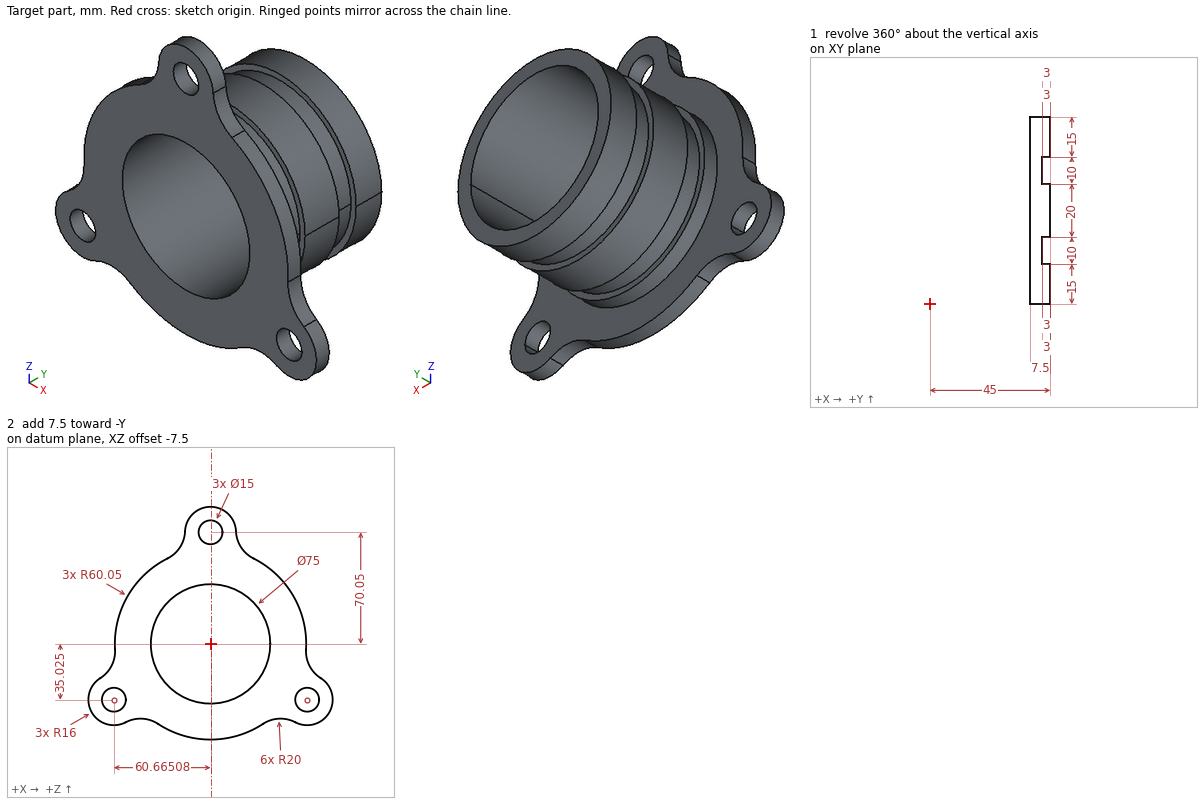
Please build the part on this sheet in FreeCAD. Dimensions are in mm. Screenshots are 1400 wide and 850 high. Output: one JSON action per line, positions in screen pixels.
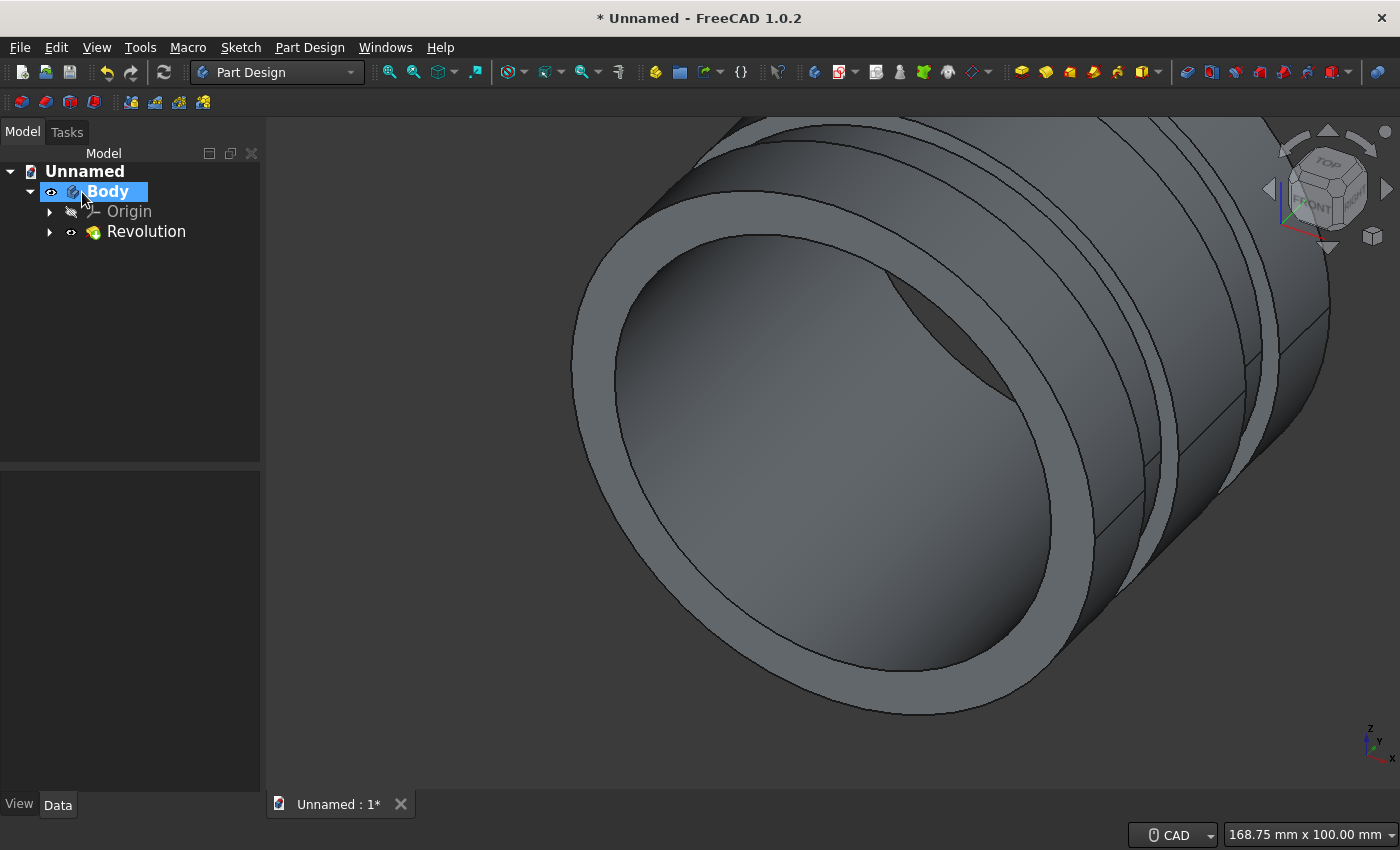
{"action": "left_click", "coordinate": [390, 72]}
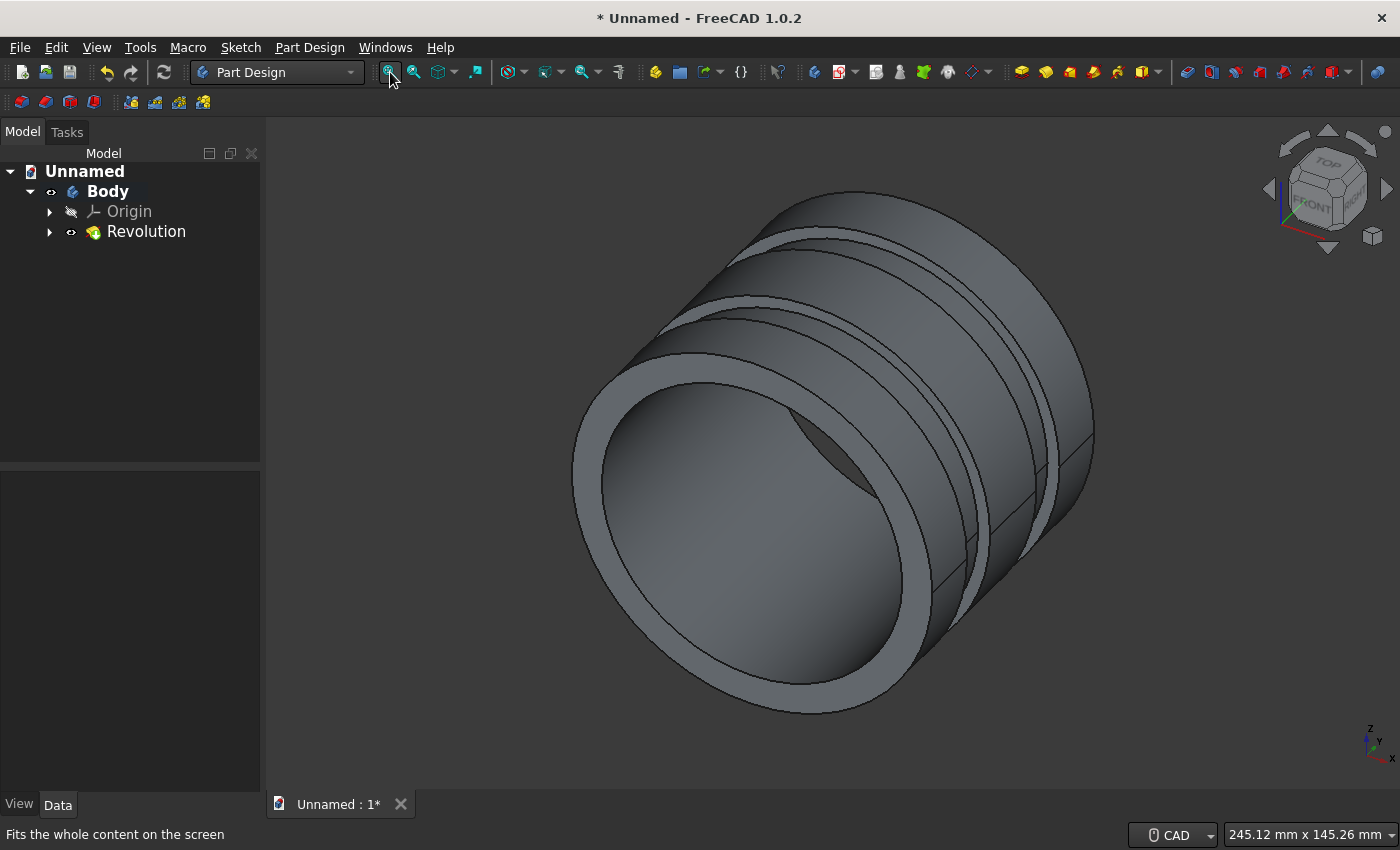
{"action": "left_click", "coordinate": [50, 212]}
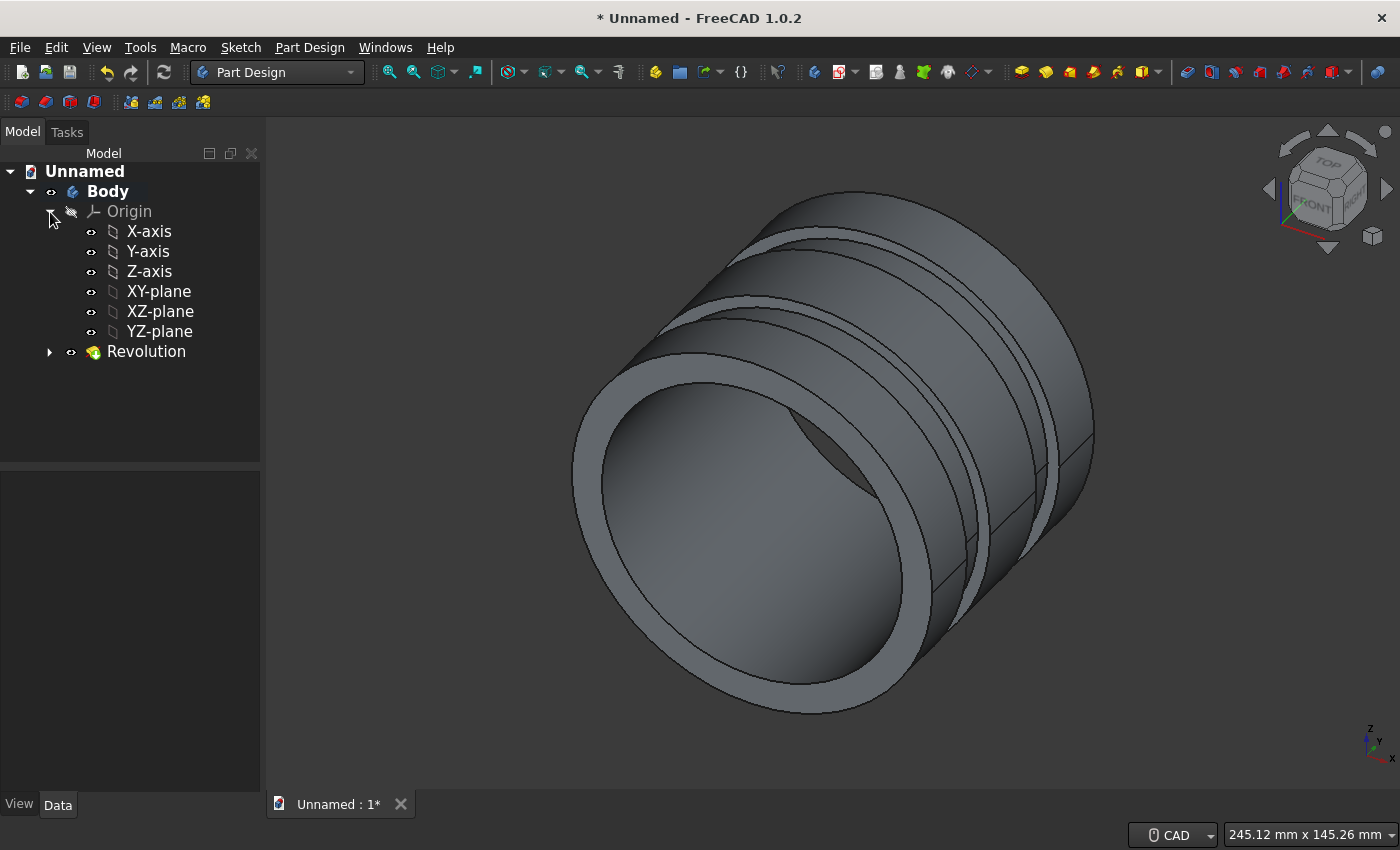
{"action": "left_click", "coordinate": [136, 312]}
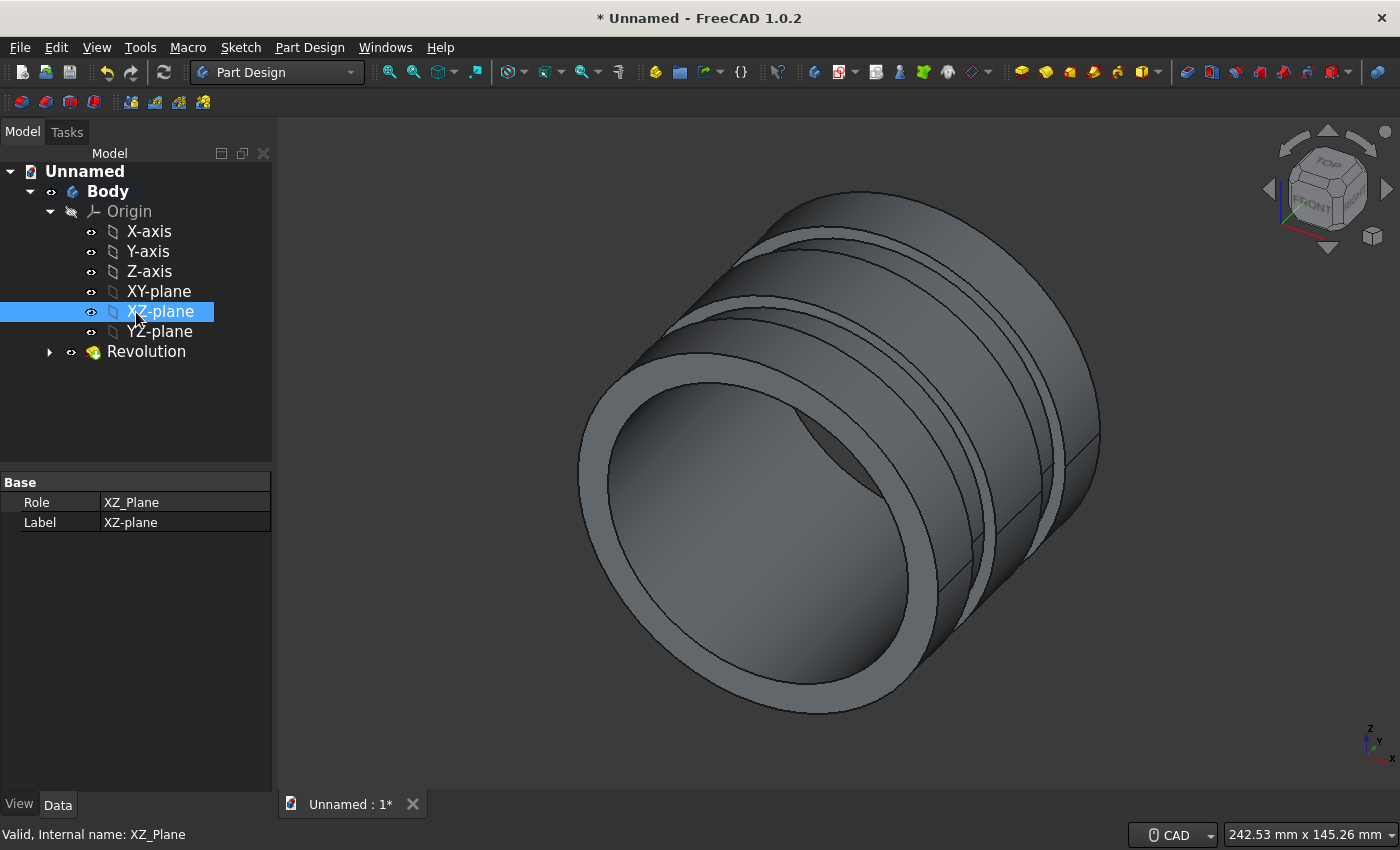
{"action": "left_click", "coordinate": [972, 72]}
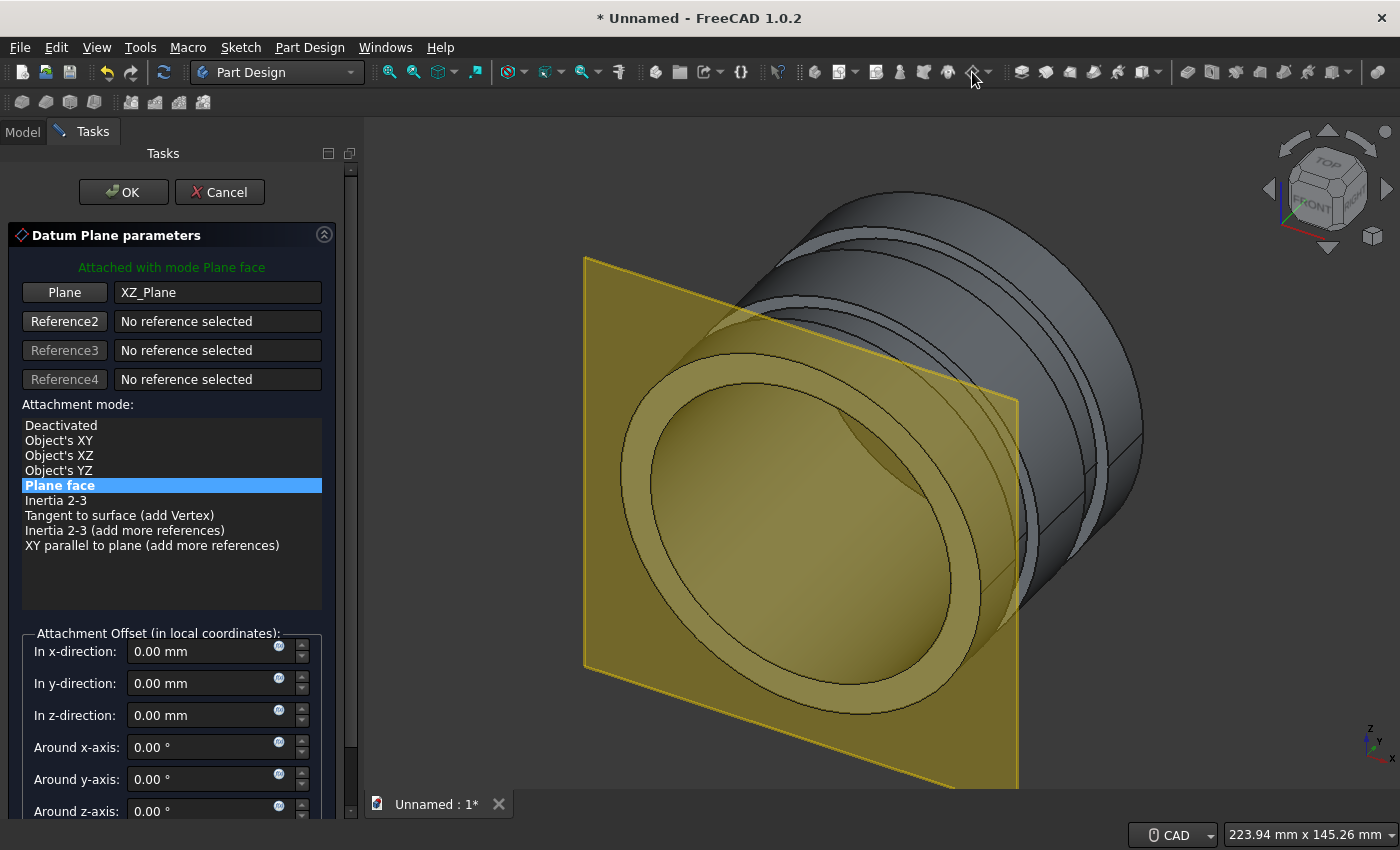
{"action": "triple_click", "coordinate": [210, 715]}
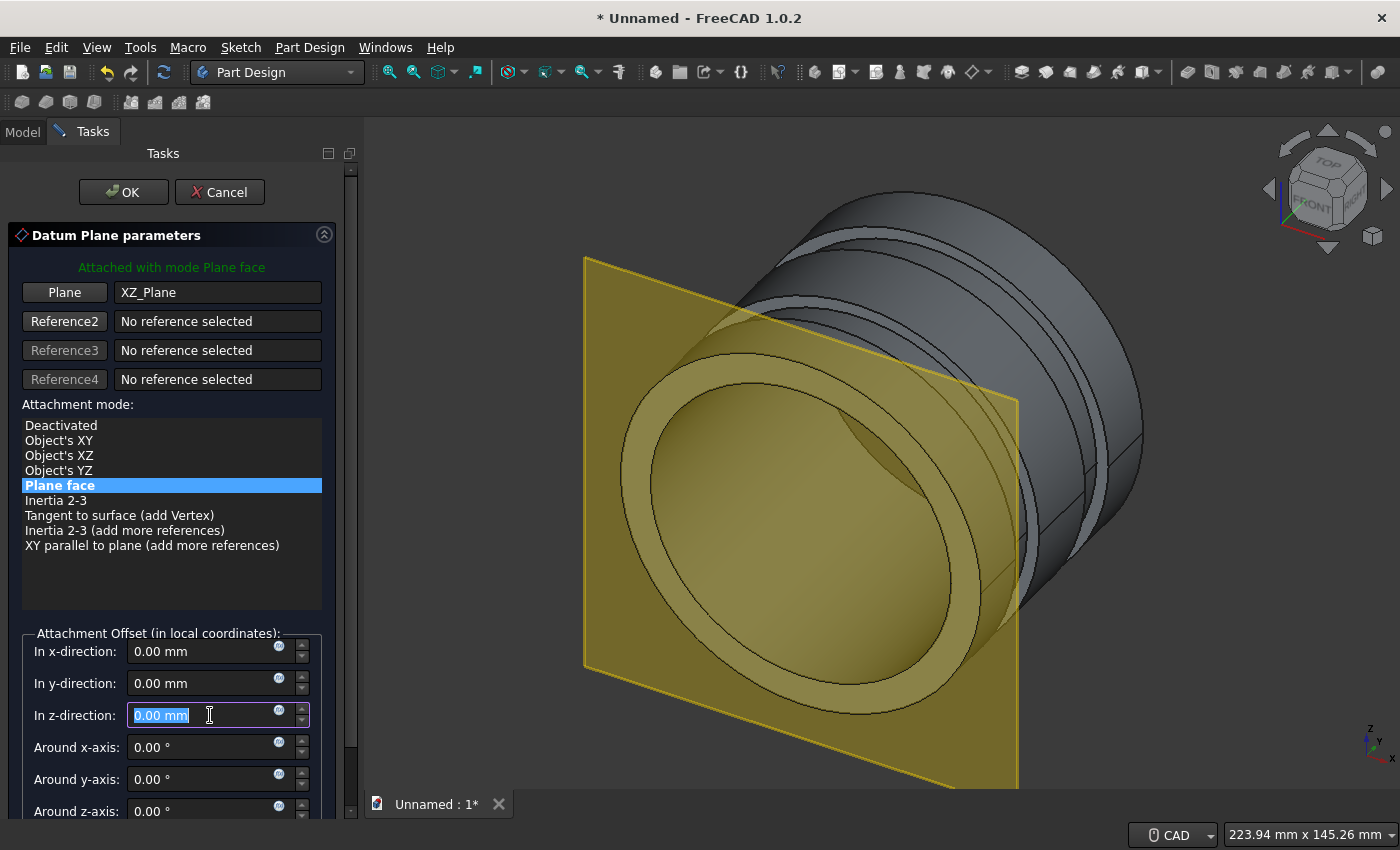
{"action": "type", "text": "-7.5"}
{"action": "key", "text": "Tab"}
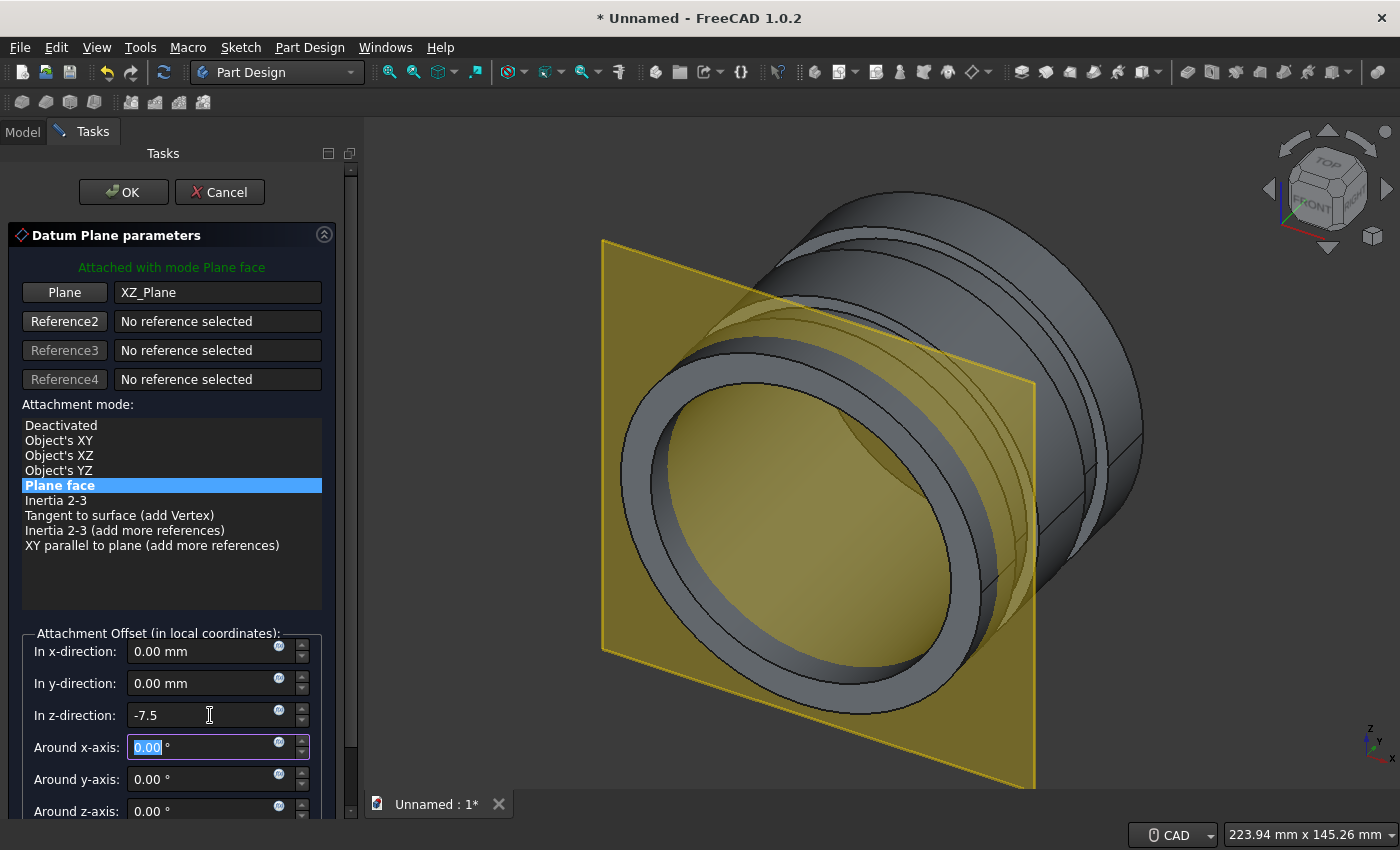
{"action": "left_click", "coordinate": [124, 192]}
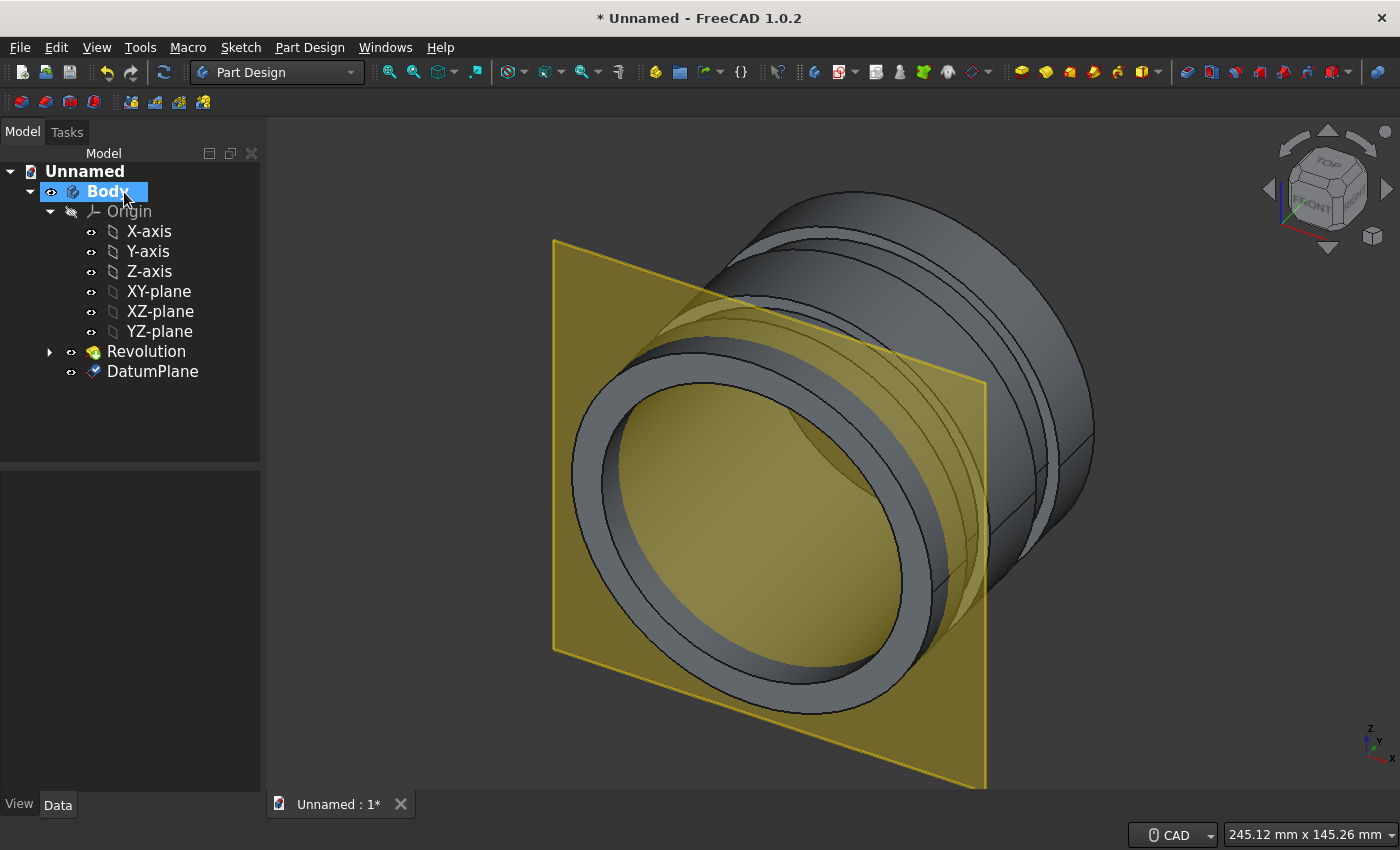
{"action": "left_click", "coordinate": [116, 372]}